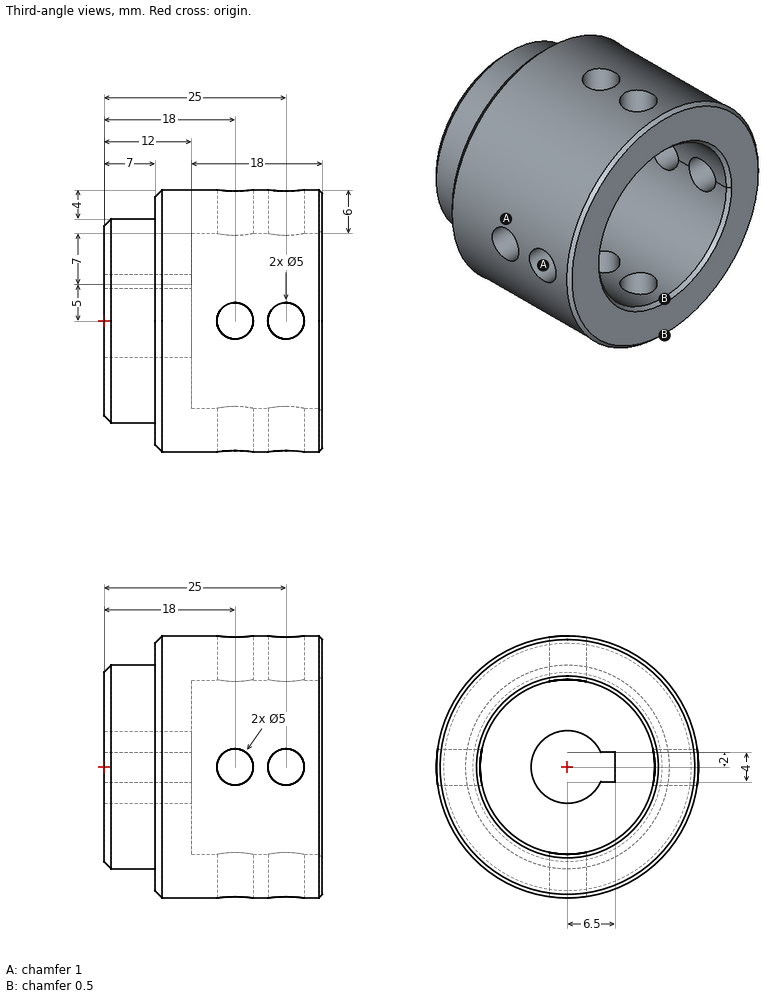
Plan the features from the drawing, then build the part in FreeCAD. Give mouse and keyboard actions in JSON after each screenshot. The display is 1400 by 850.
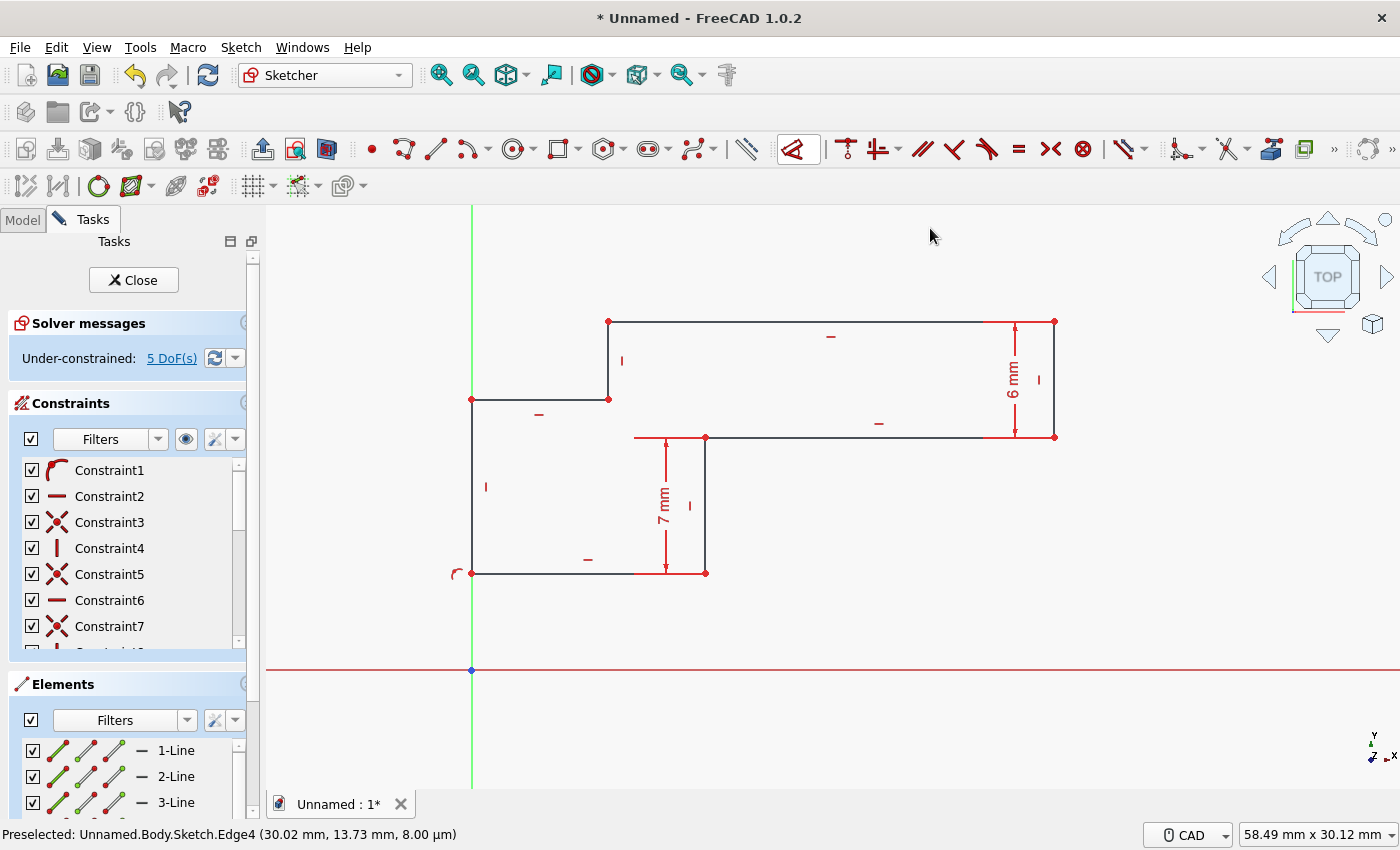
{"action": "left_click", "coordinate": [608, 345]}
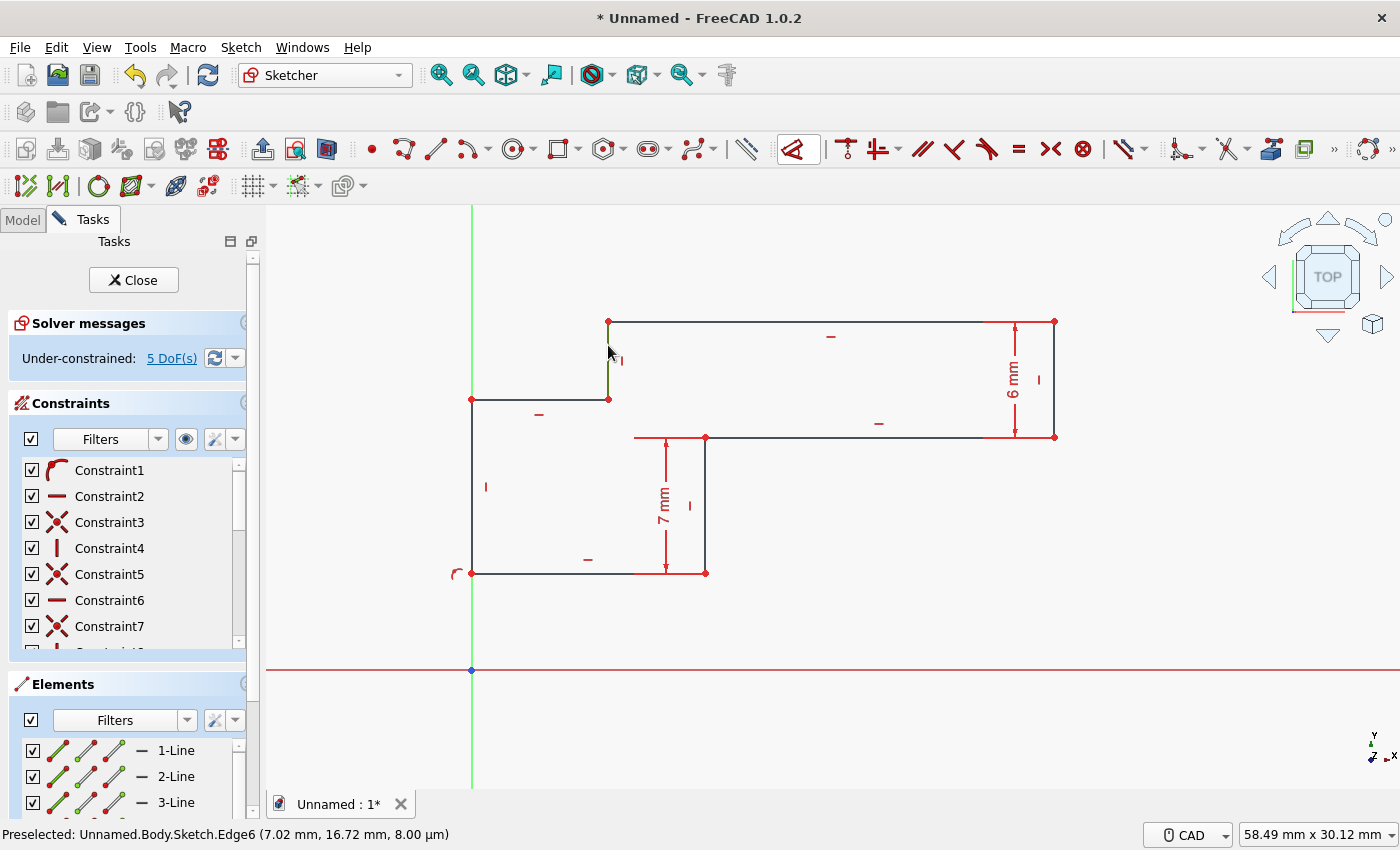
{"action": "left_click", "coordinate": [814, 150]}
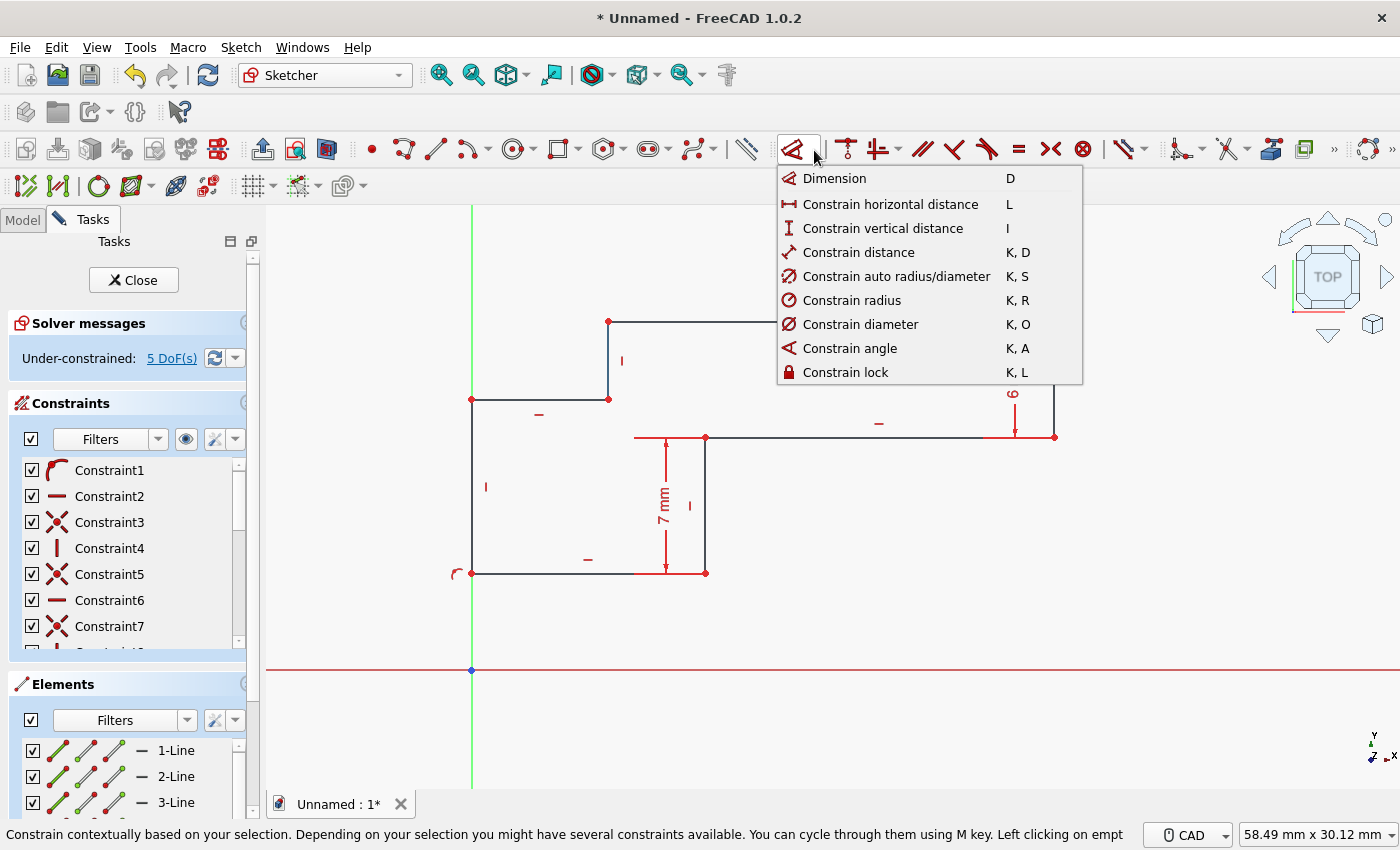
{"action": "left_click", "coordinate": [930, 228]}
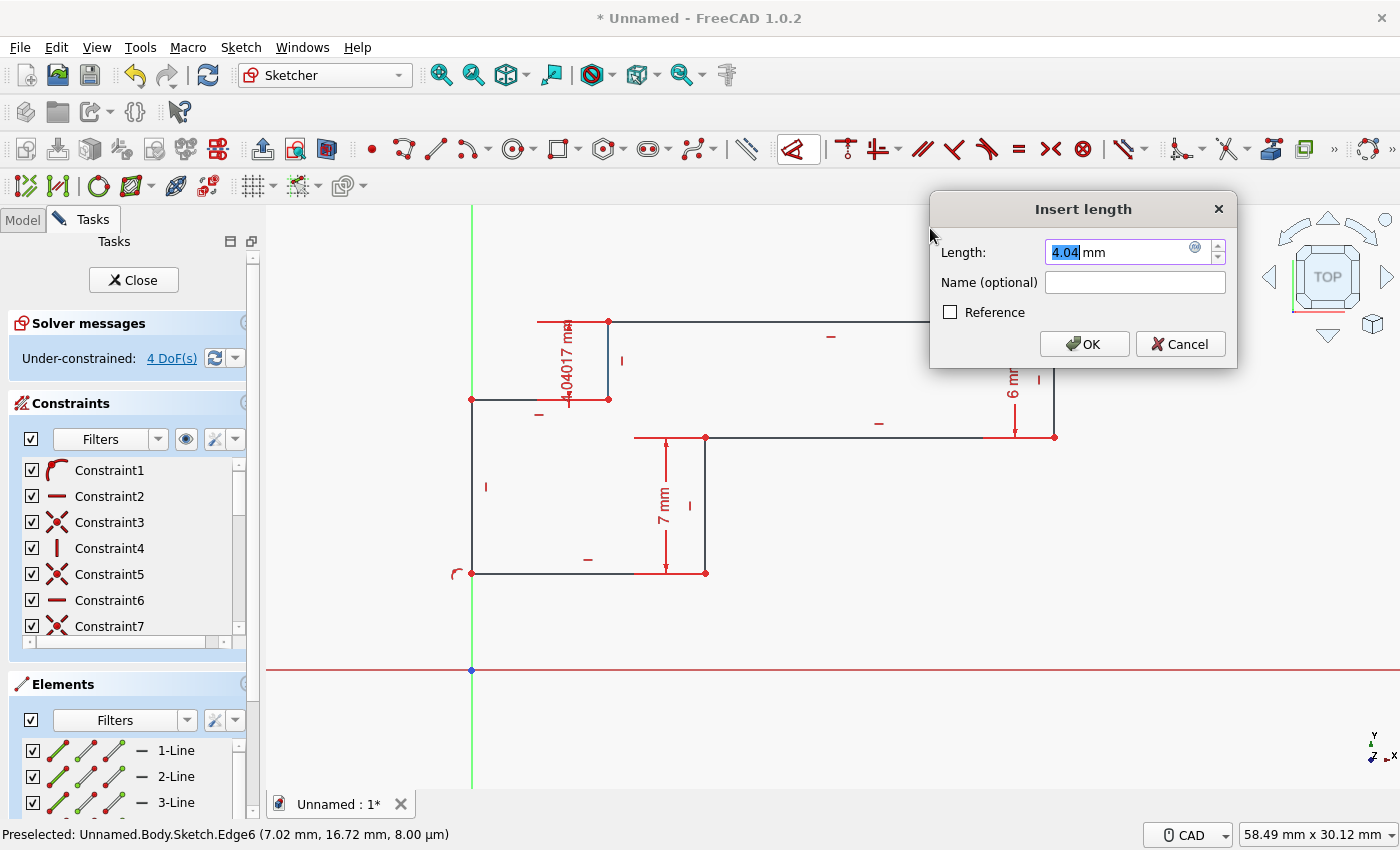
{"action": "type", "text": "4"}
{"action": "key", "text": "Return"}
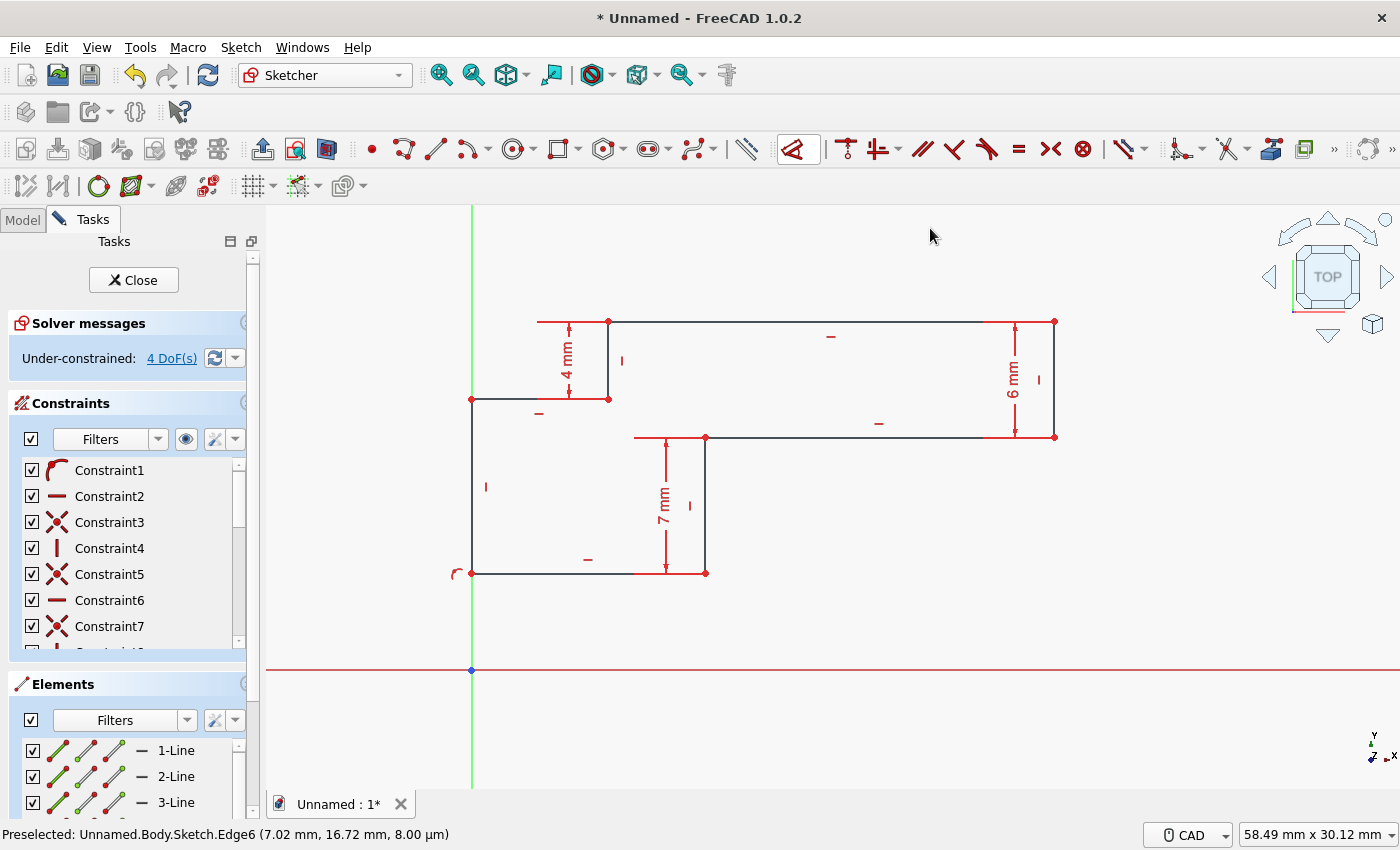
{"action": "left_click", "coordinate": [567, 399]}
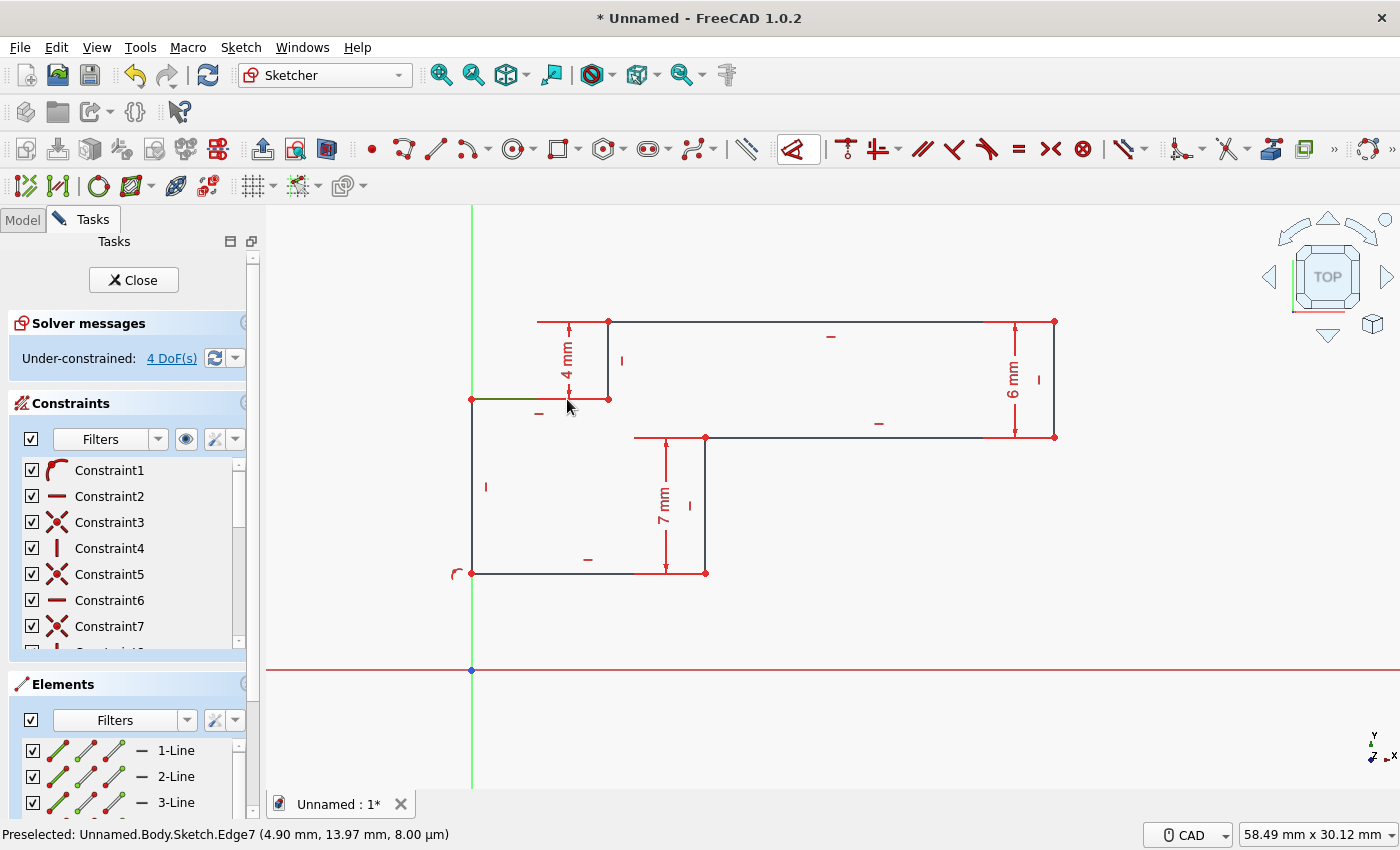
{"action": "key", "text": "l"}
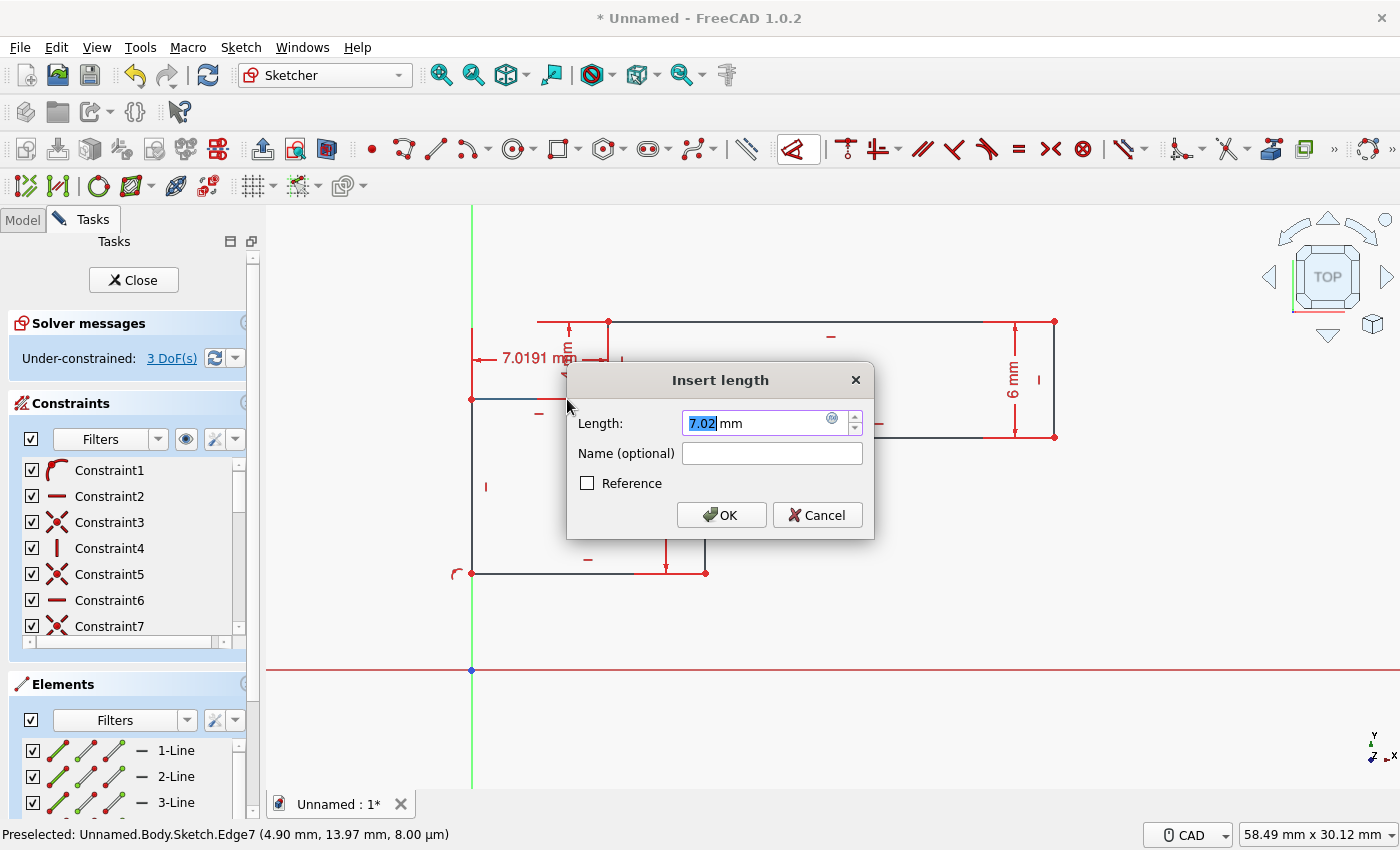
{"action": "type", "text": "7"}
{"action": "key", "text": "Return"}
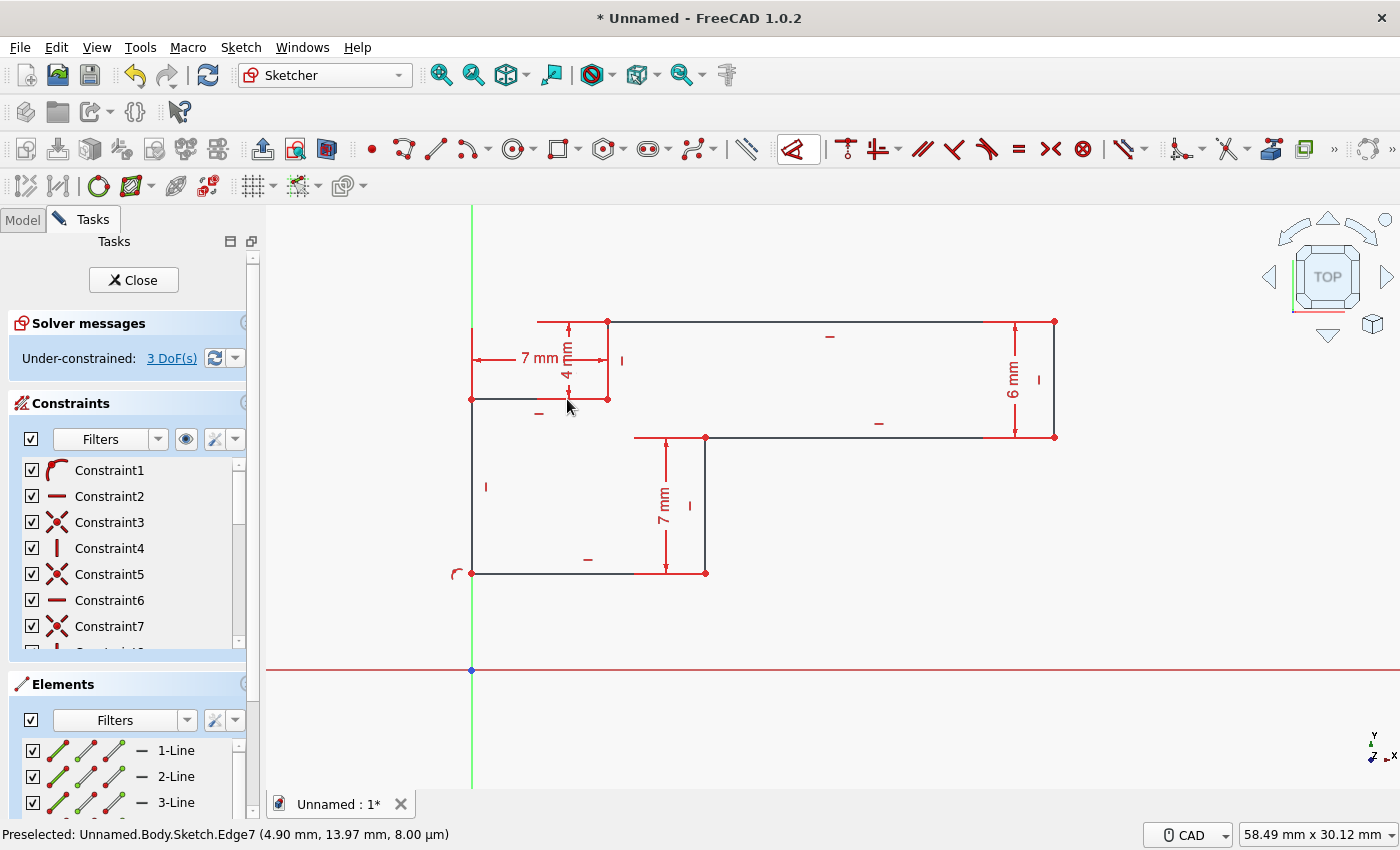
{"action": "left_click", "coordinate": [542, 574]}